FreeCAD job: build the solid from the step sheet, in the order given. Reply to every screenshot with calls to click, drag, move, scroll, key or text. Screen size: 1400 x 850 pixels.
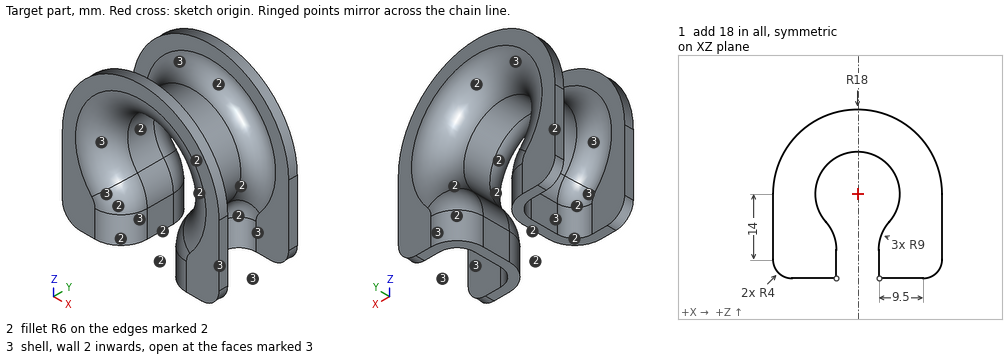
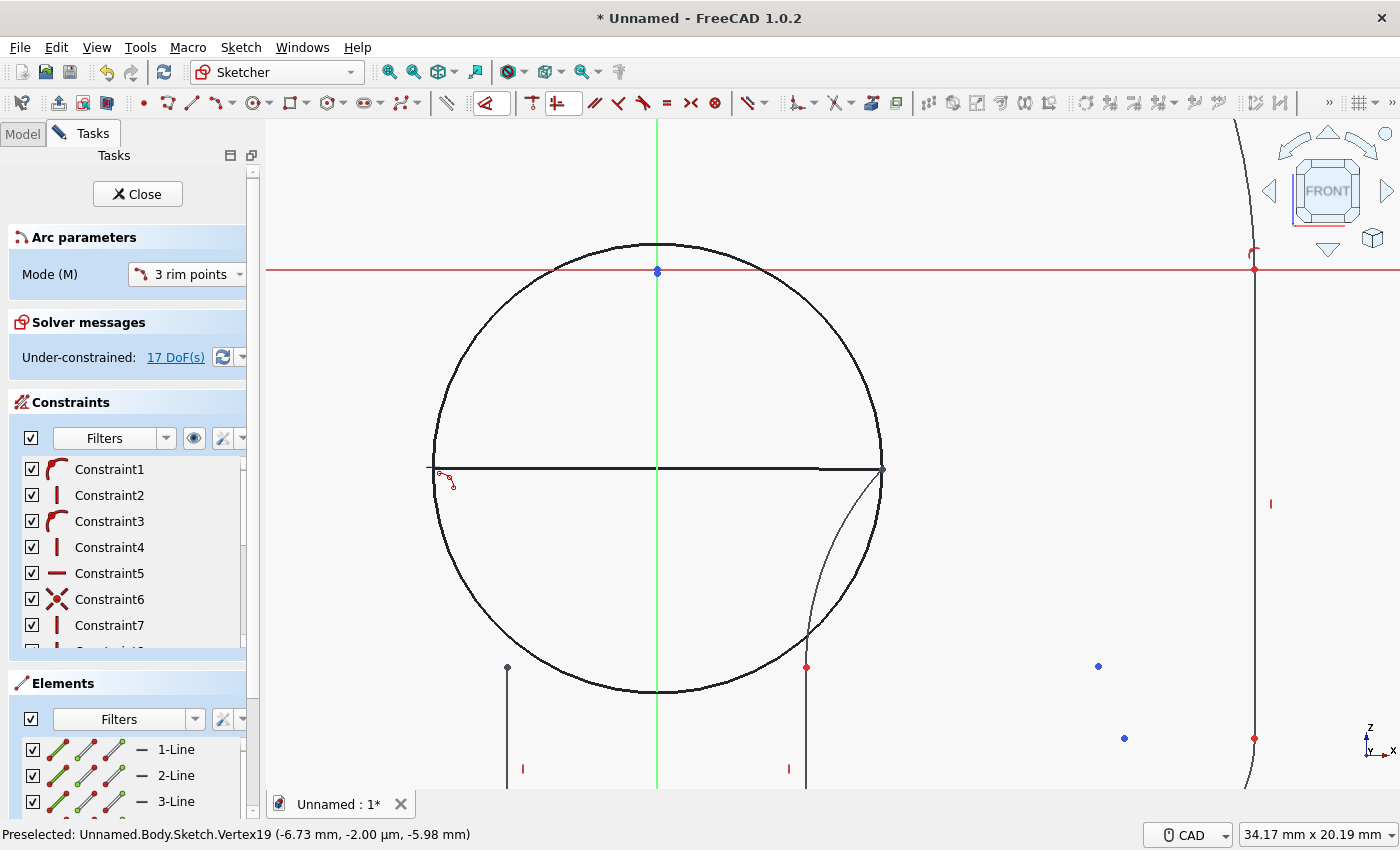
scroll(827, 561, down, 5)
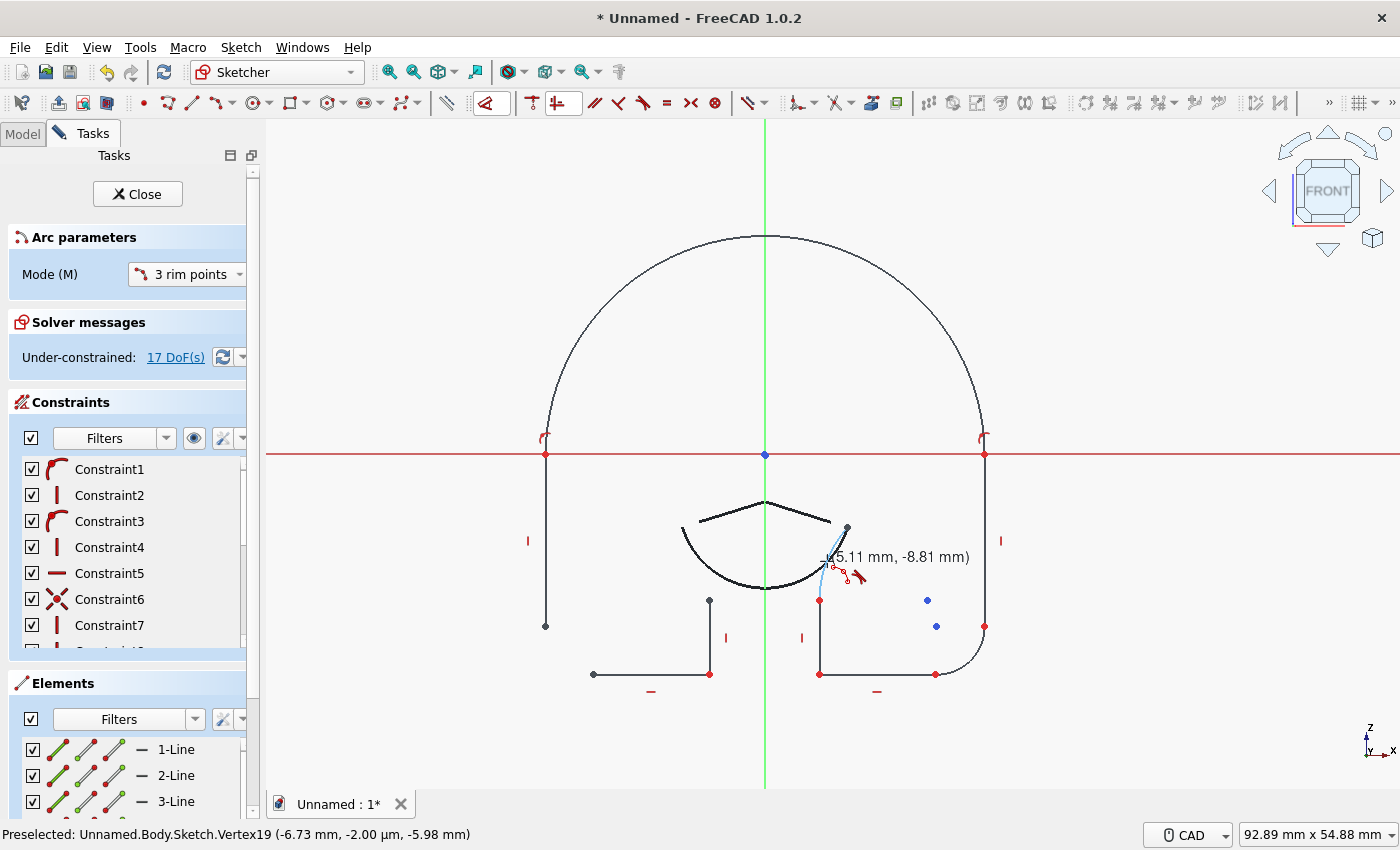
click(814, 356)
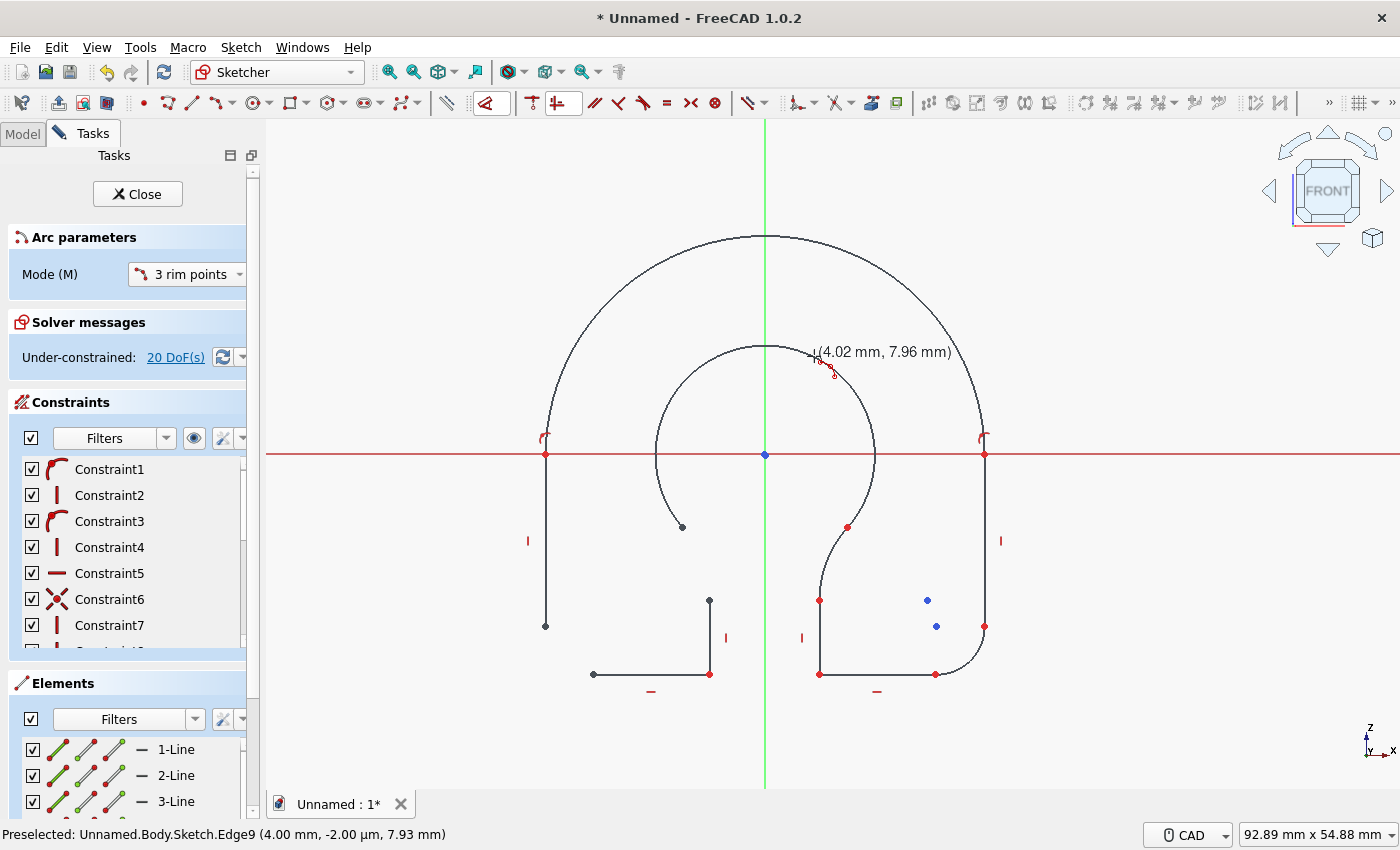
click(682, 527)
click(710, 601)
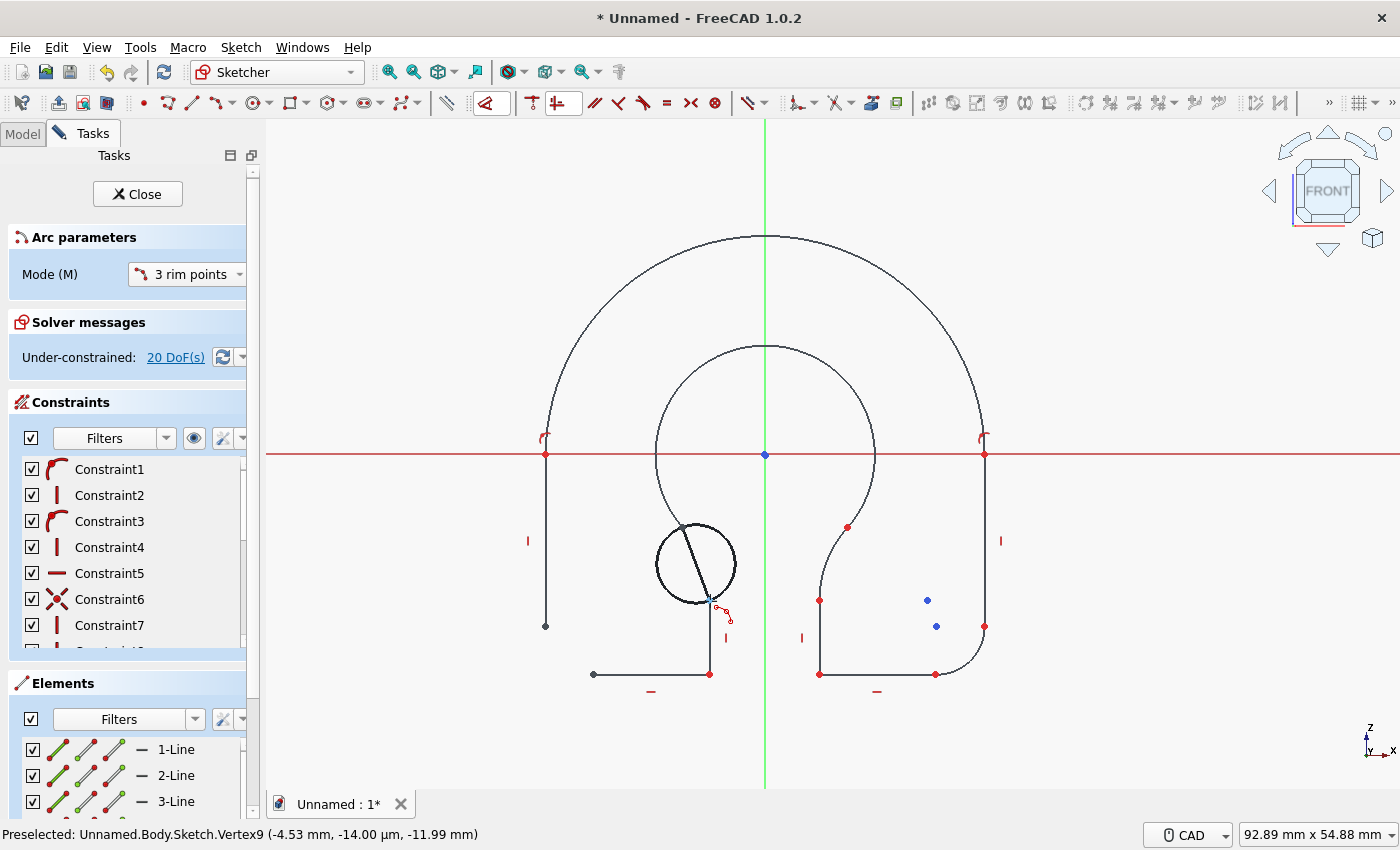
scroll(703, 561, up, 5)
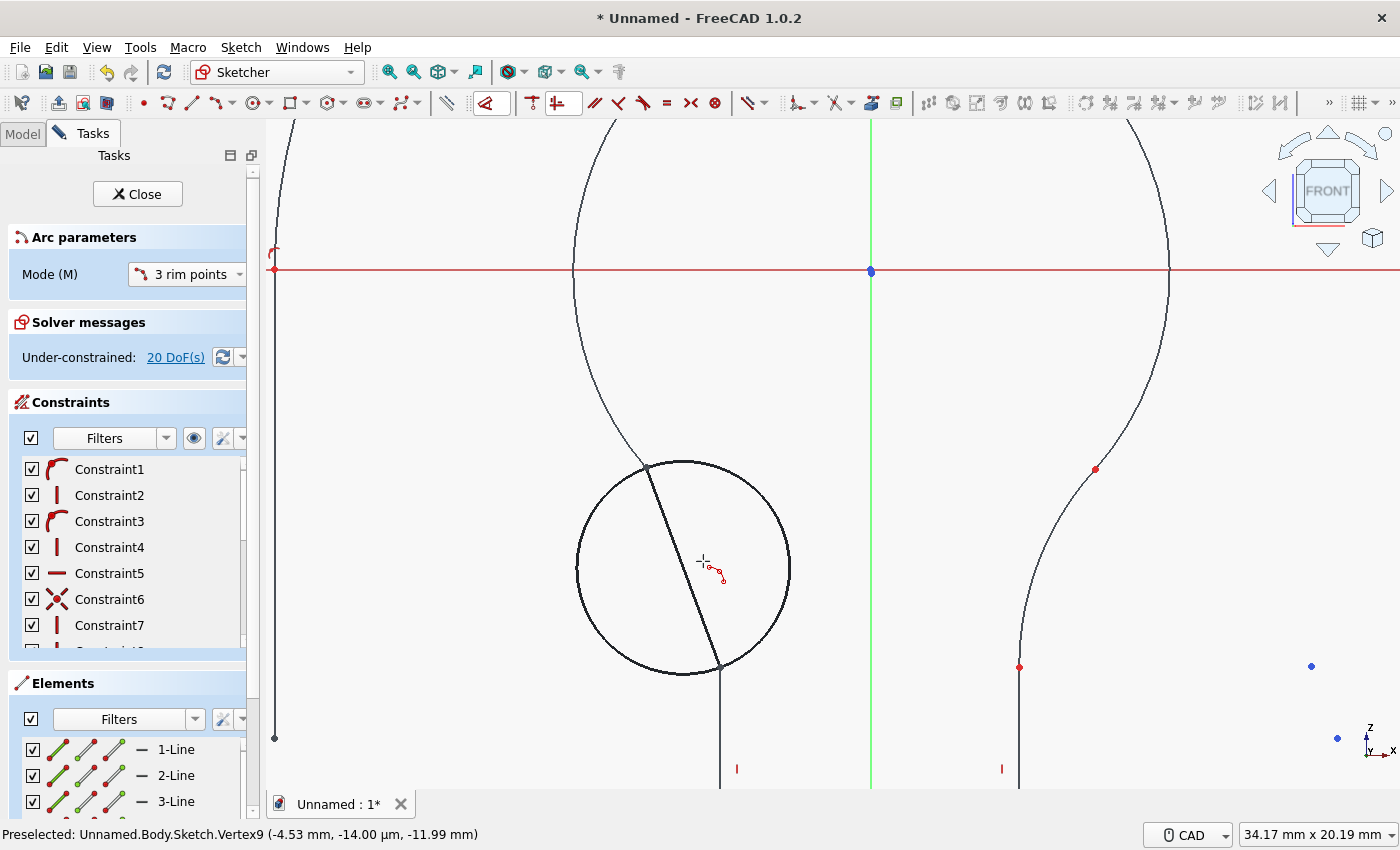
click(702, 559)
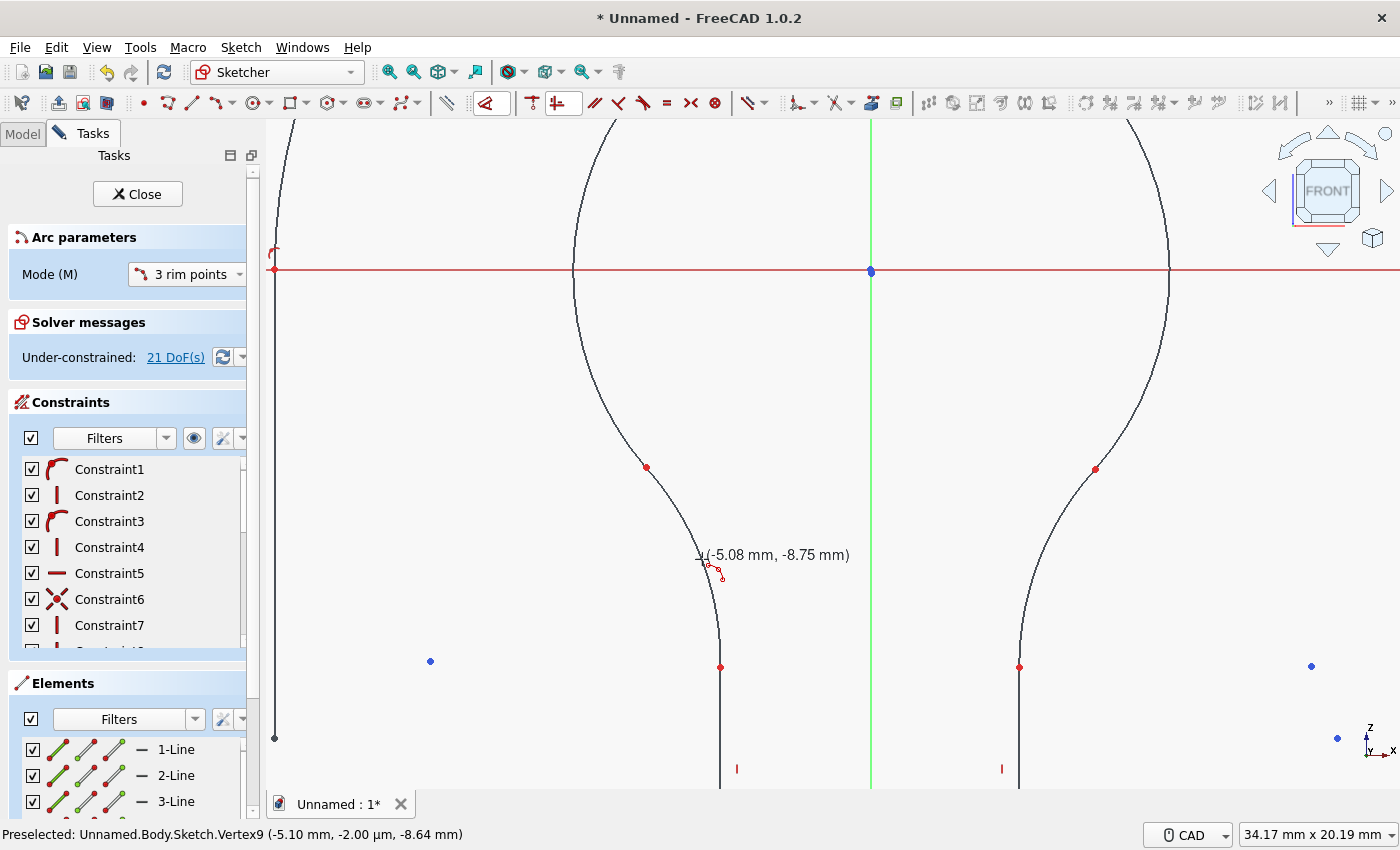
scroll(703, 561, down, 5)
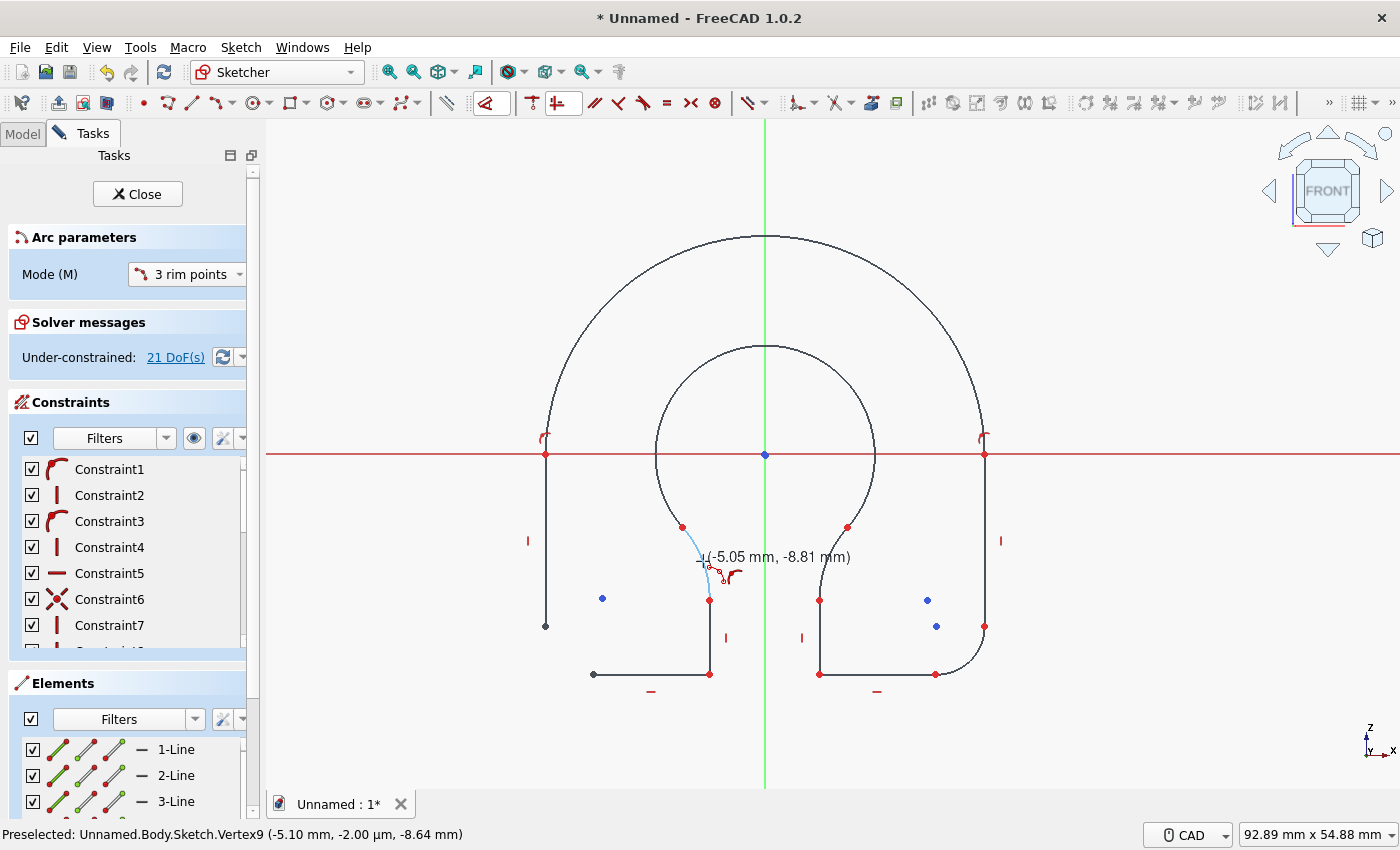
click(594, 675)
click(546, 627)
click(559, 660)
key(Escape)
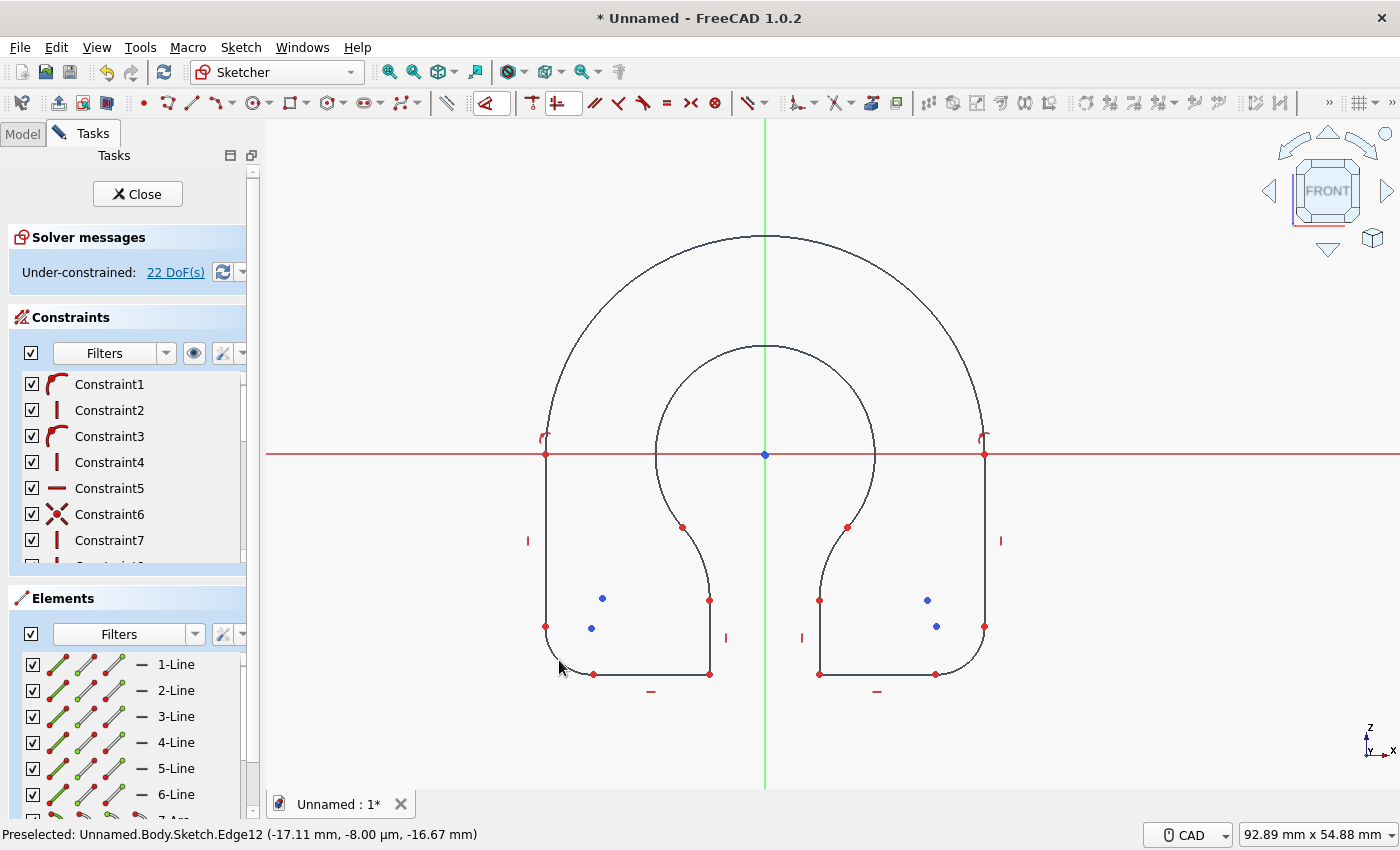
click(546, 575)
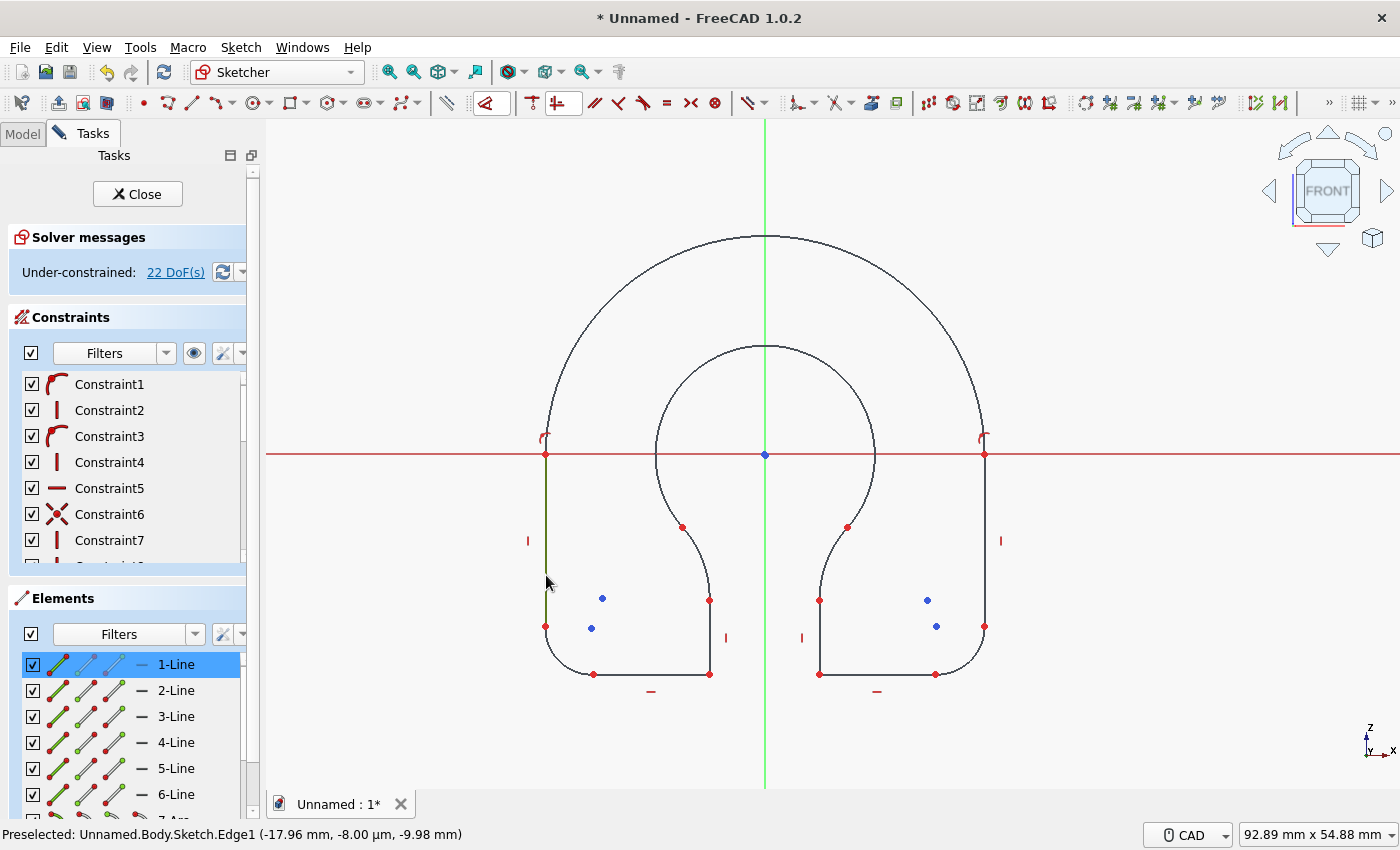
click(894, 278)